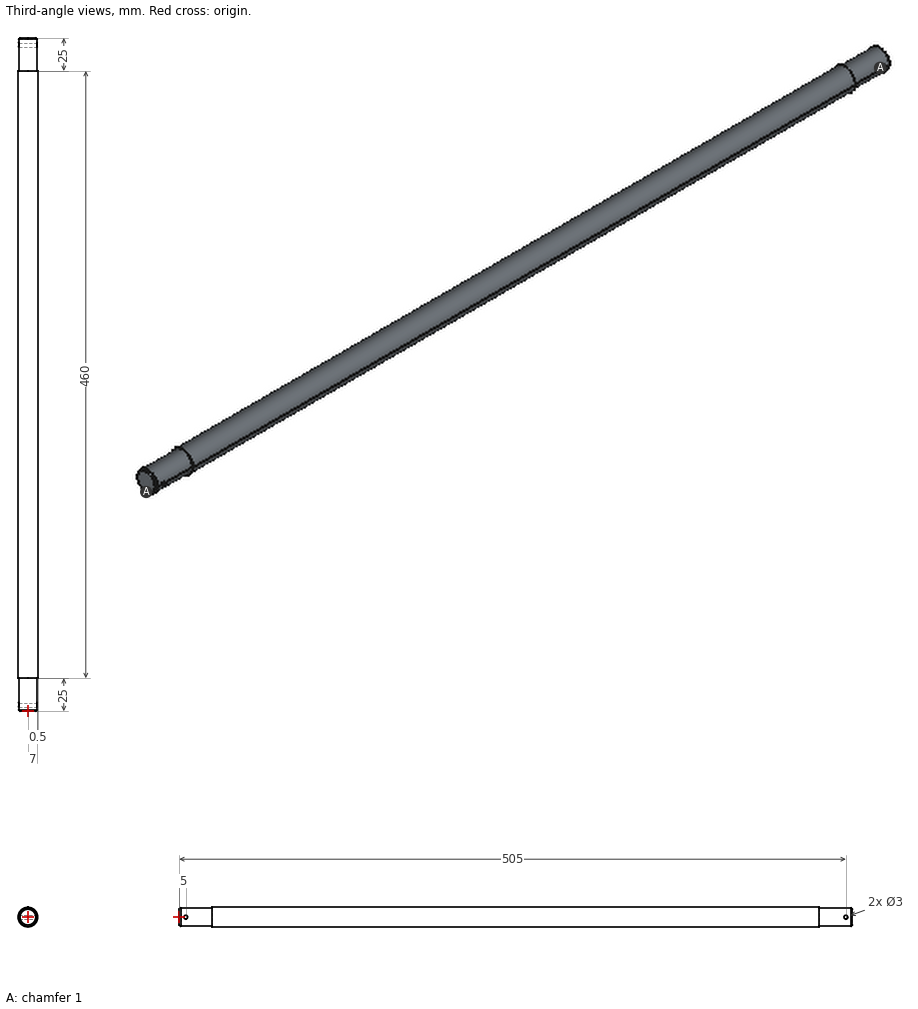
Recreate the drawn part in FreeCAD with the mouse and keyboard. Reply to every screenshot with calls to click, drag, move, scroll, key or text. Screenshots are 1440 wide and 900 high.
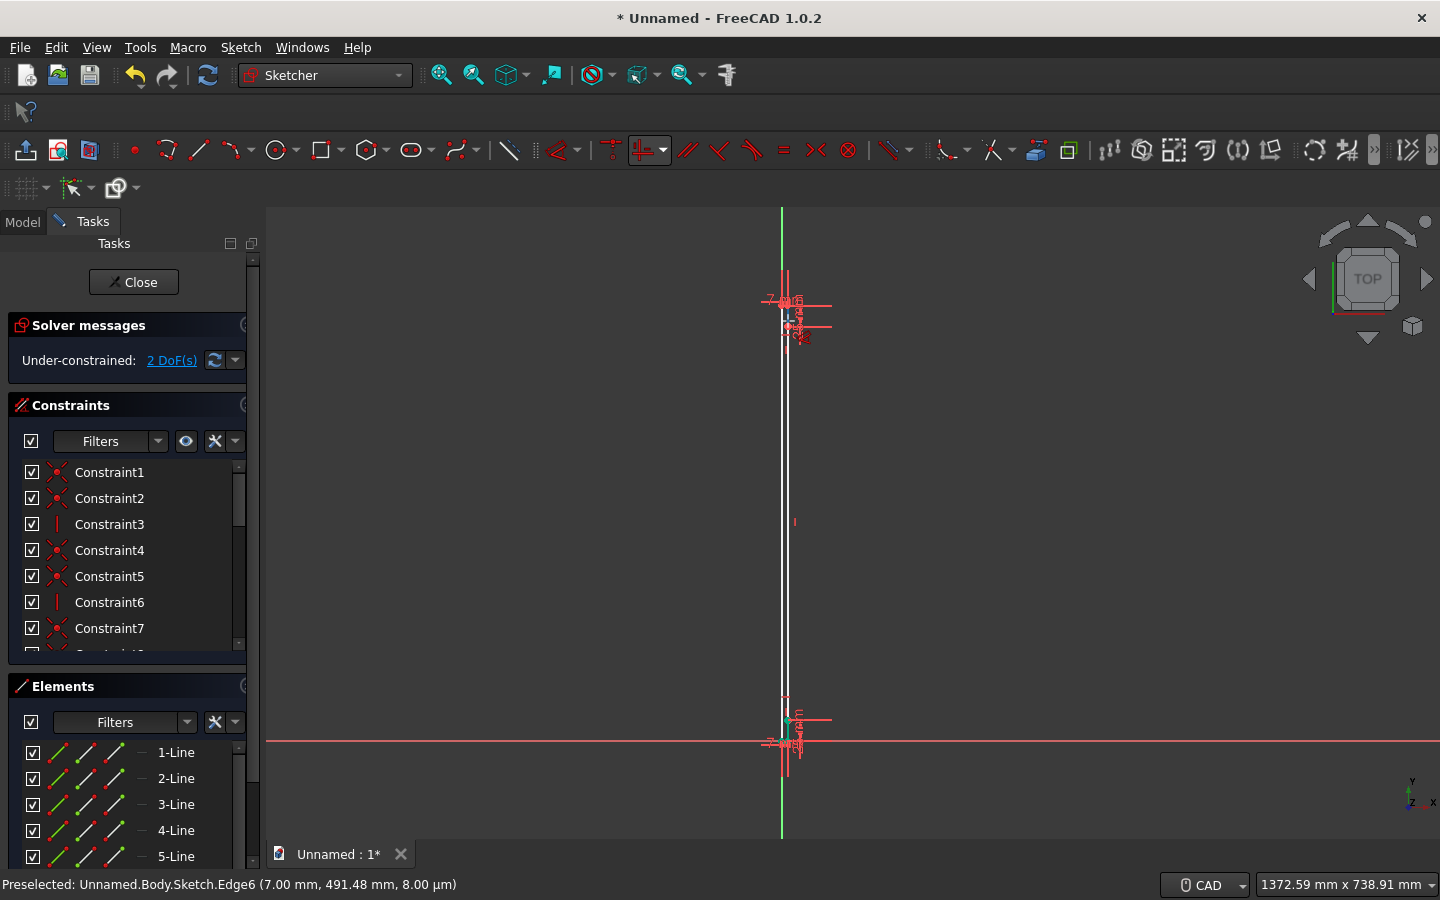
scroll(788, 720, up, 23)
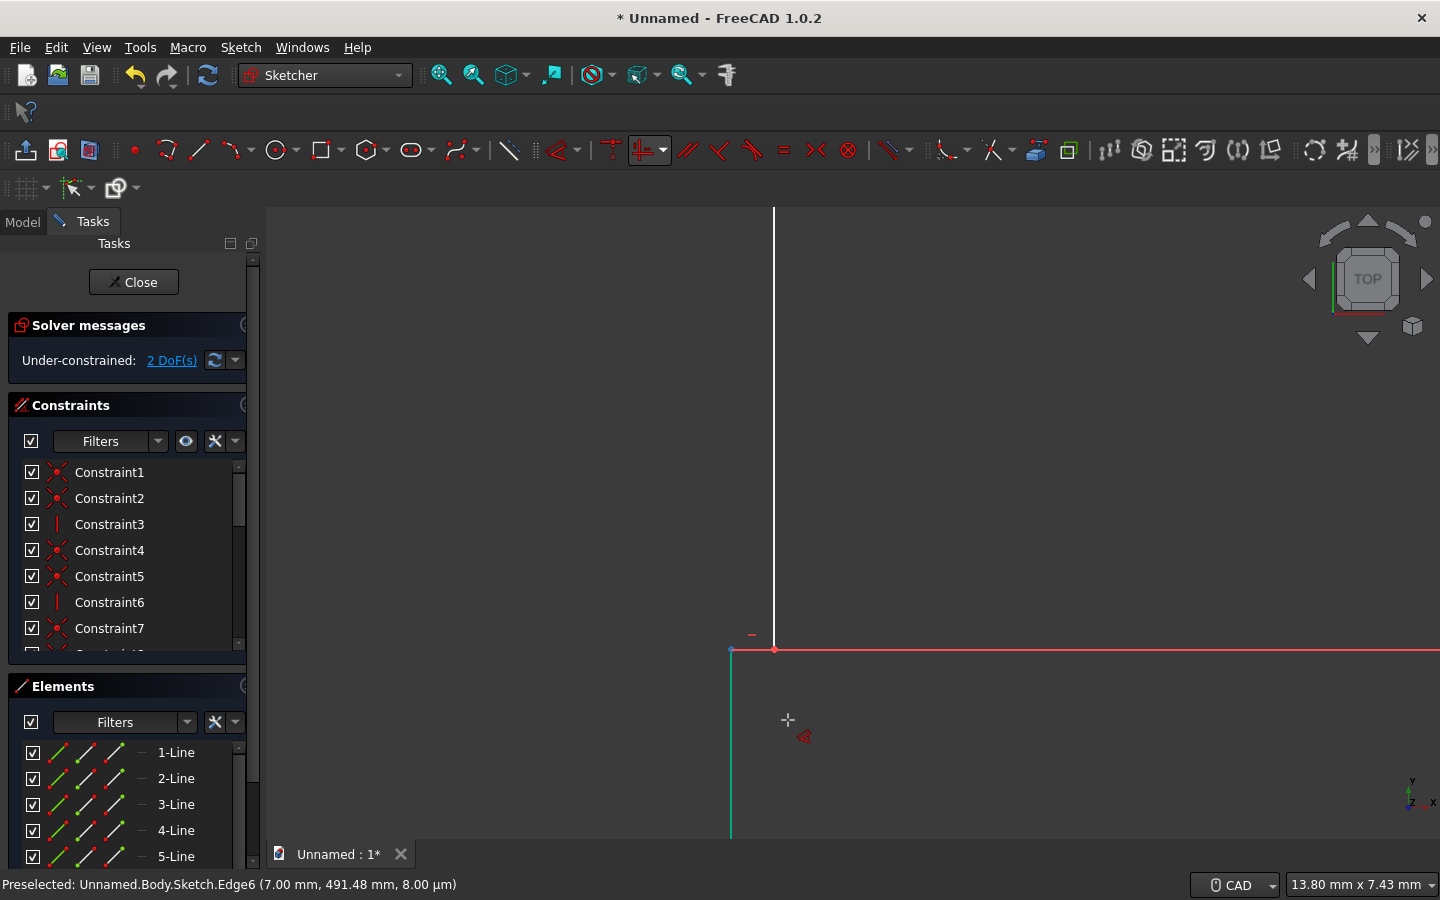
click(753, 650)
click(753, 684)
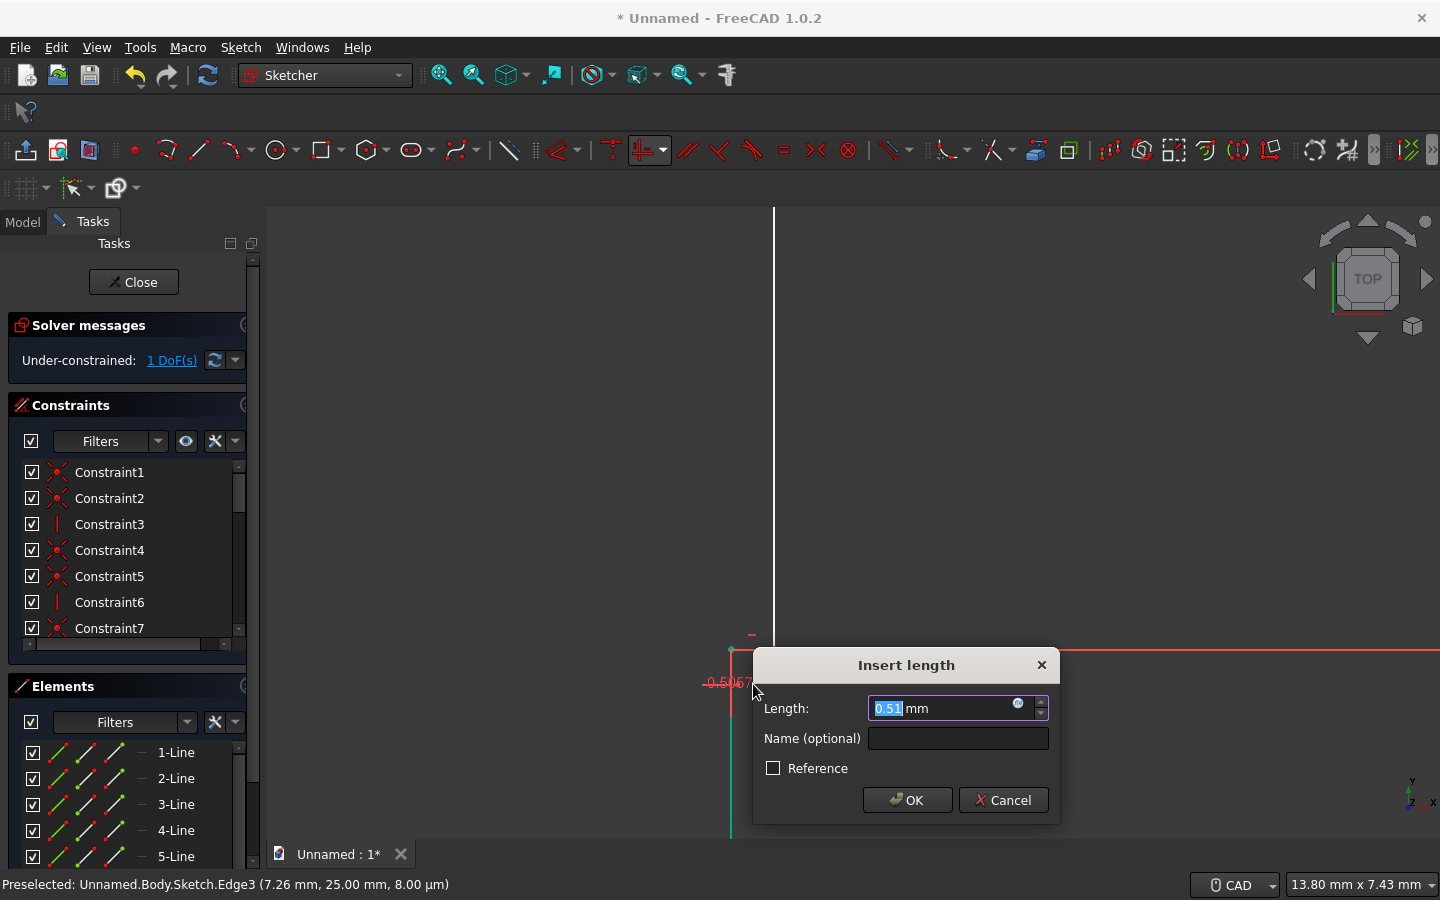
text(0.5)
key(Return)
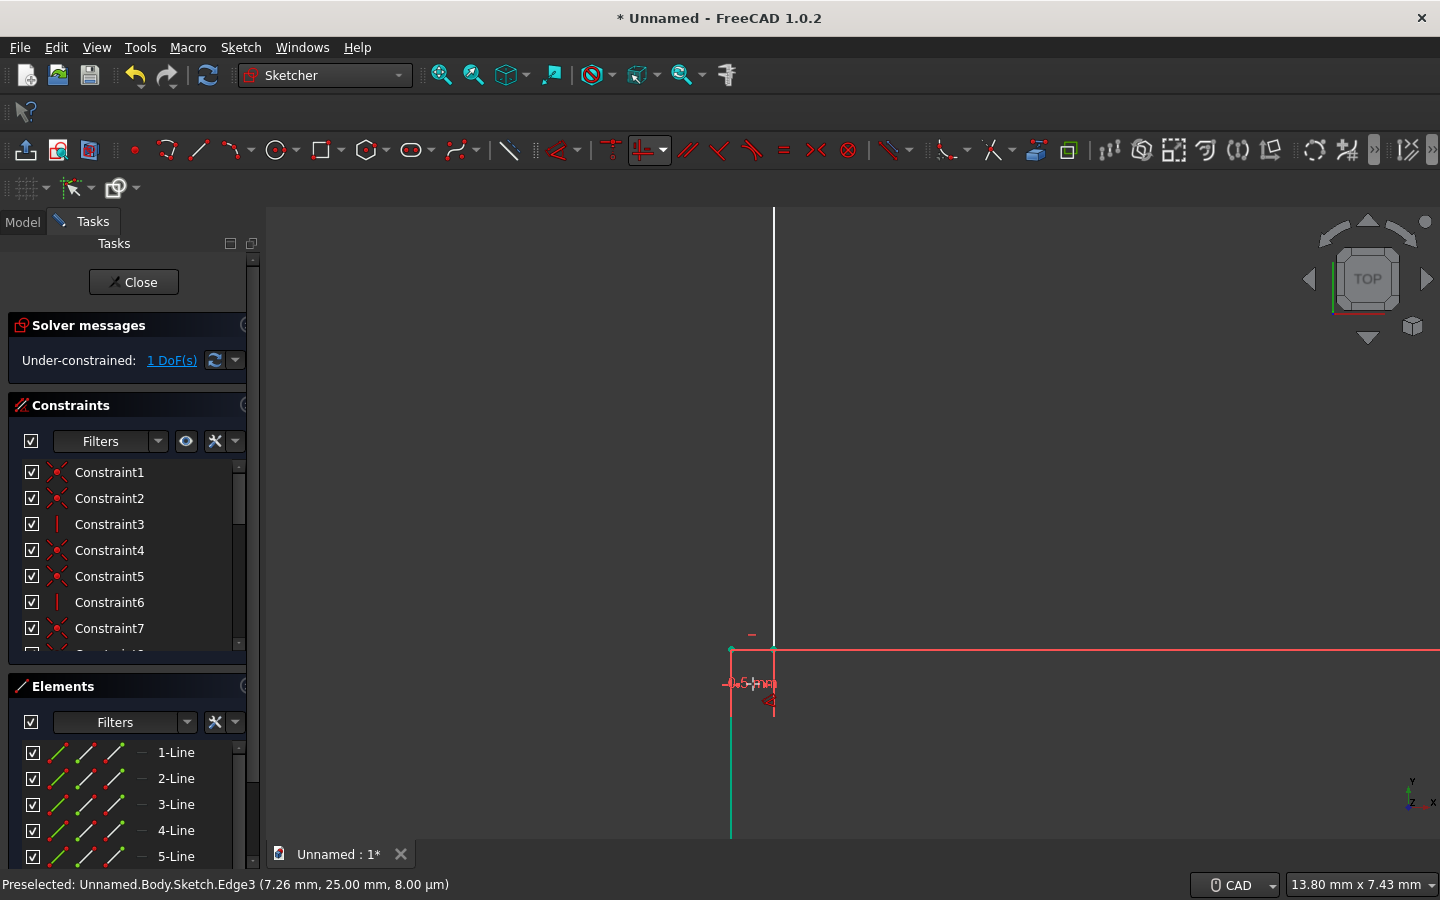
scroll(784, 523, down, 15)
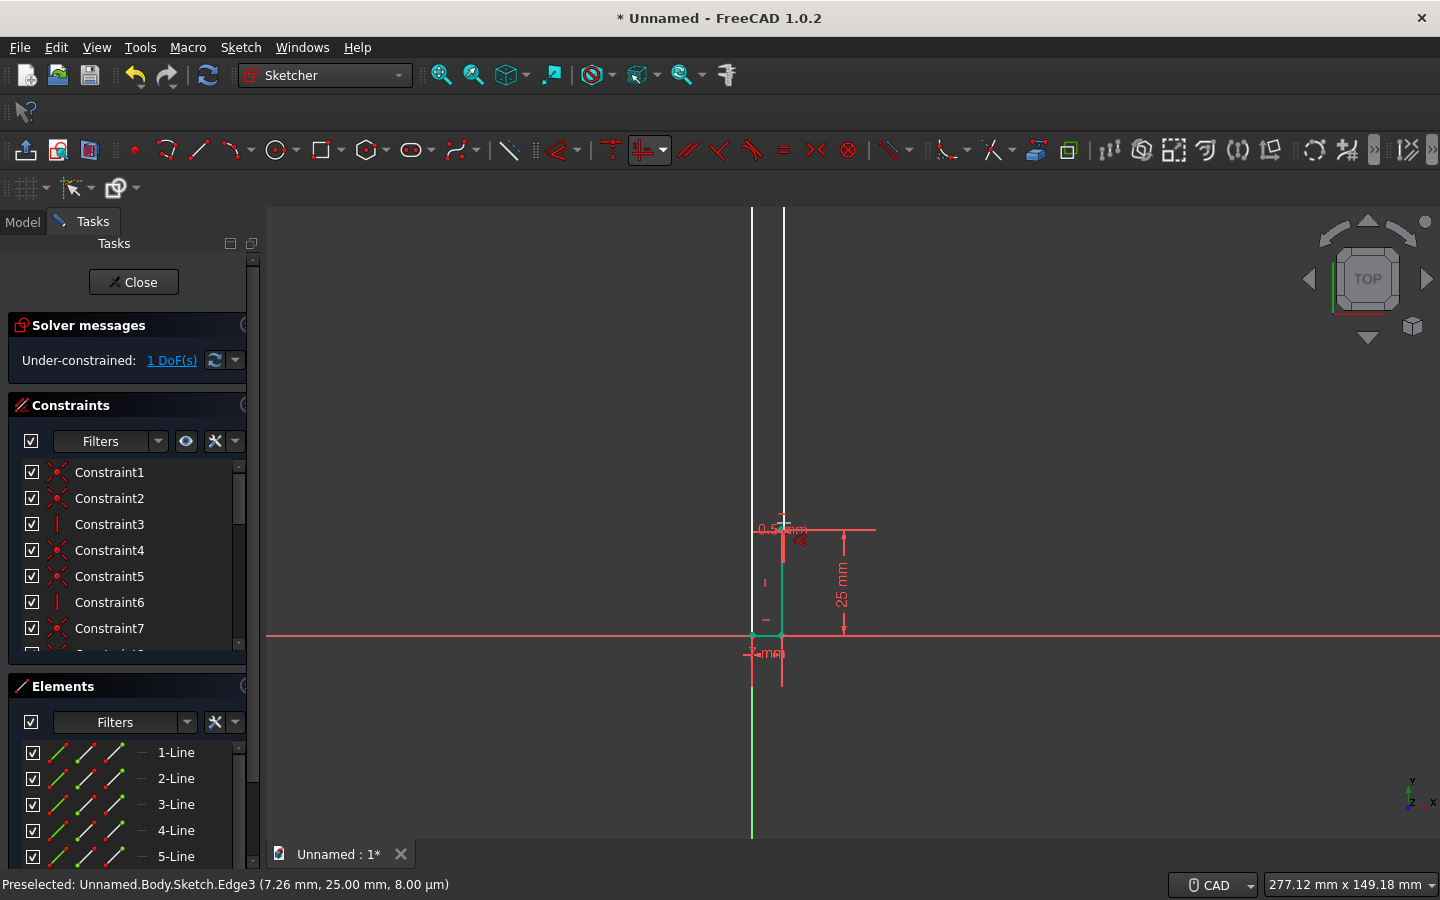
scroll(789, 768, down, 8)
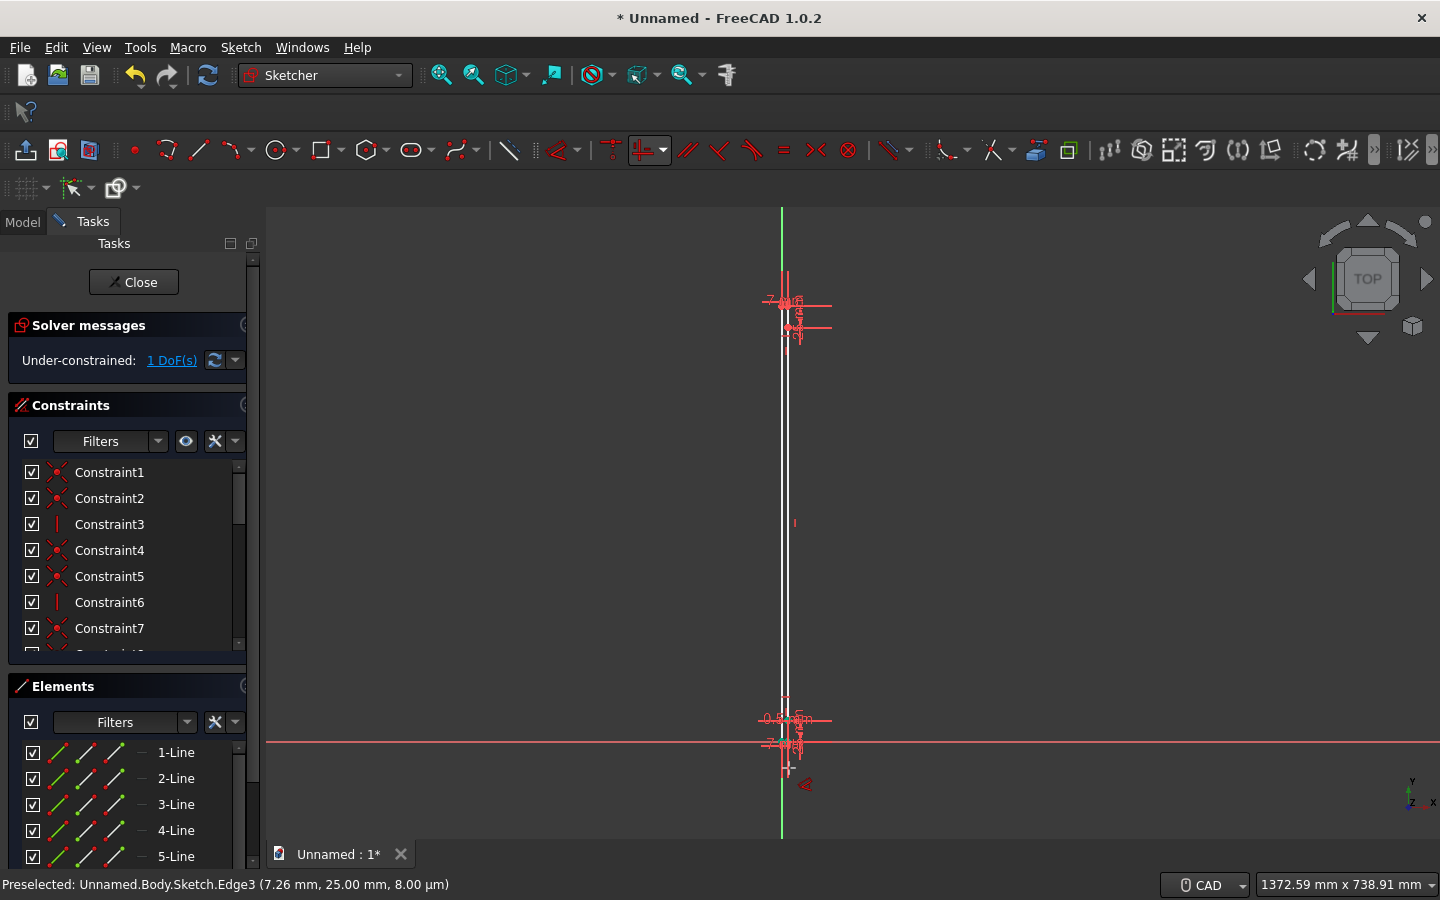
scroll(788, 603, up, 4)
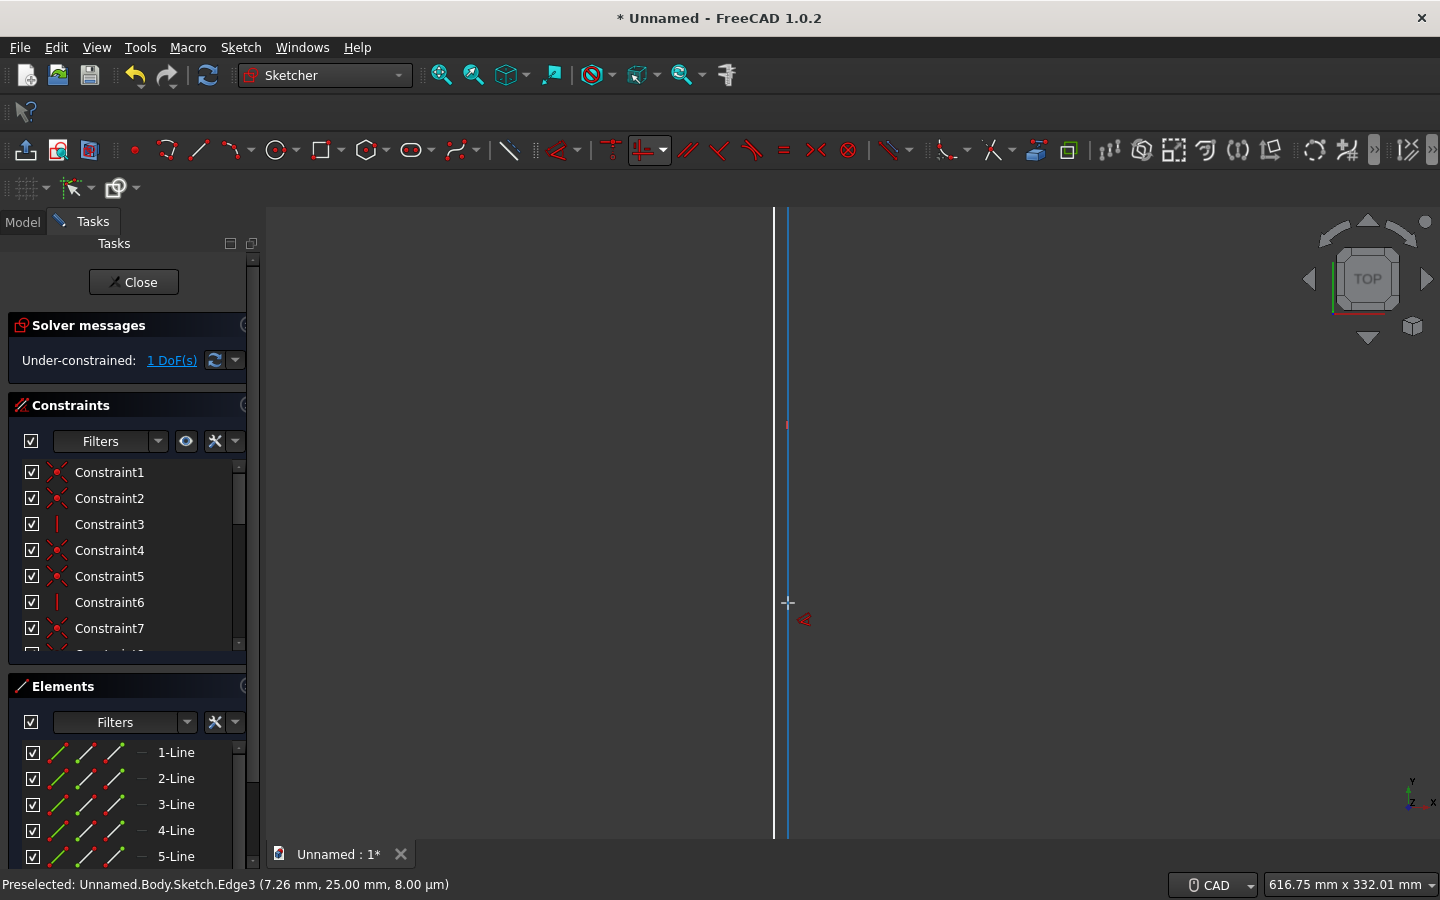
click(788, 602)
click(822, 523)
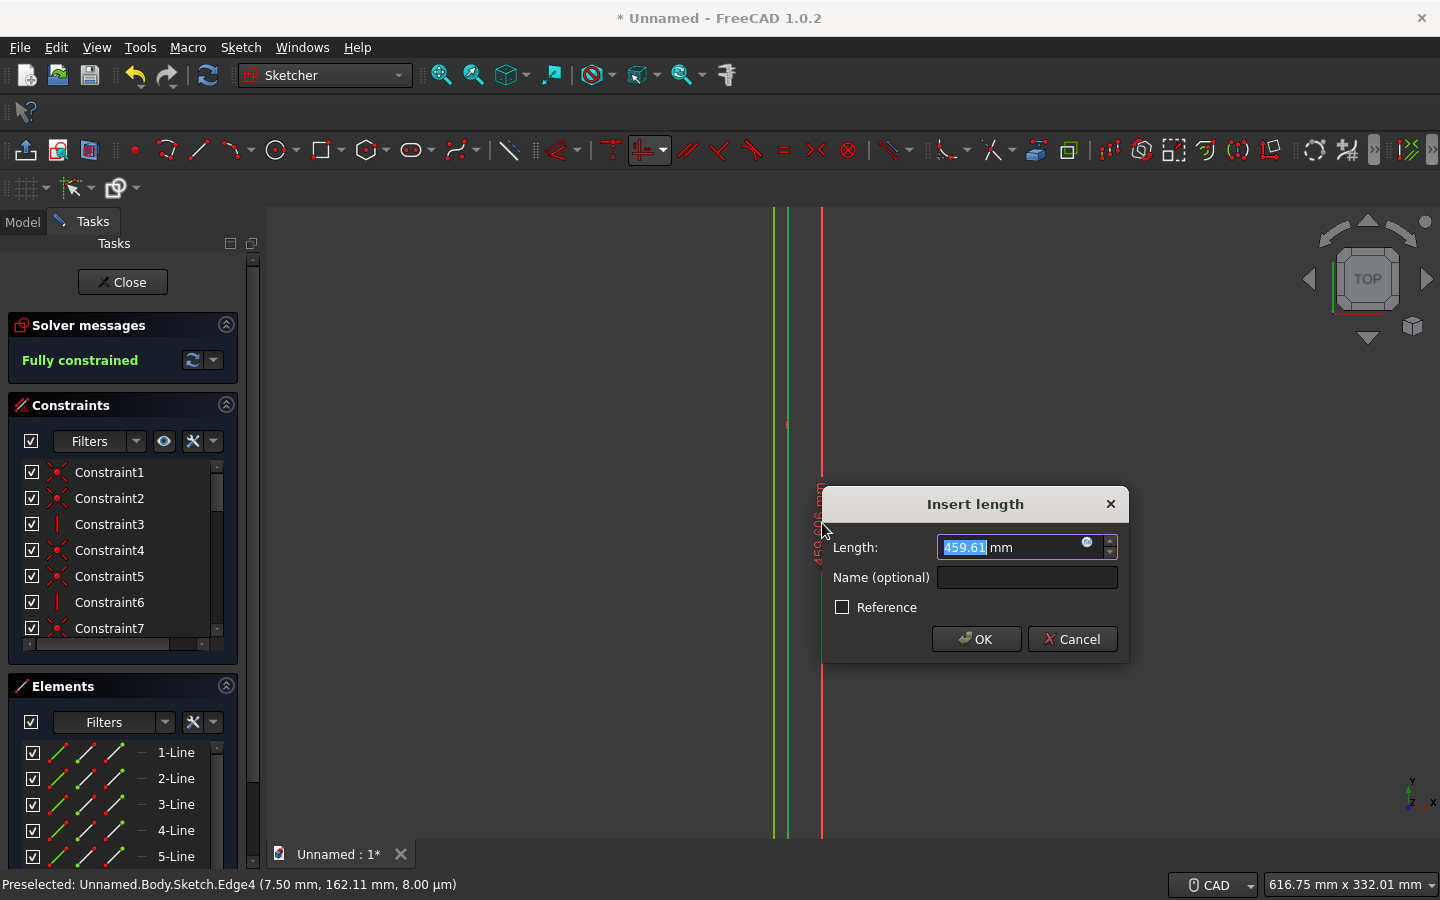
text(460)
key(Return)
key(Escape)